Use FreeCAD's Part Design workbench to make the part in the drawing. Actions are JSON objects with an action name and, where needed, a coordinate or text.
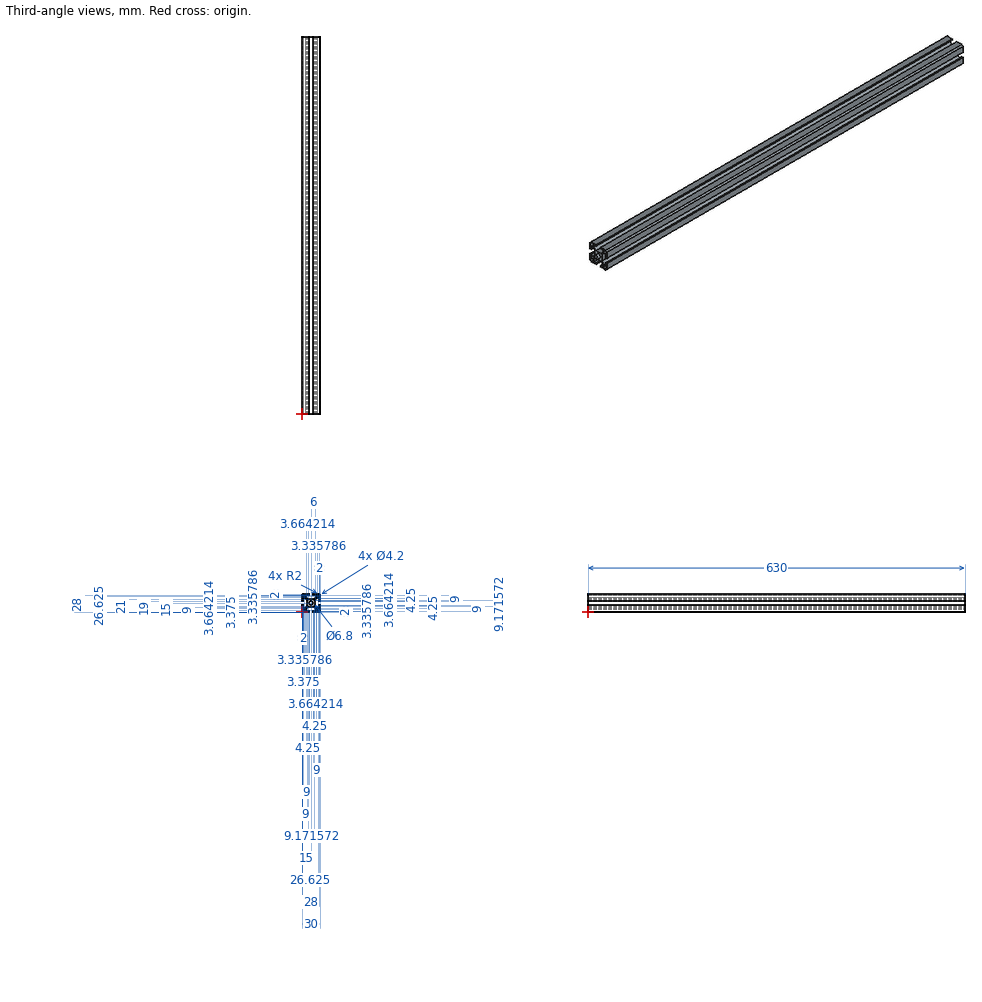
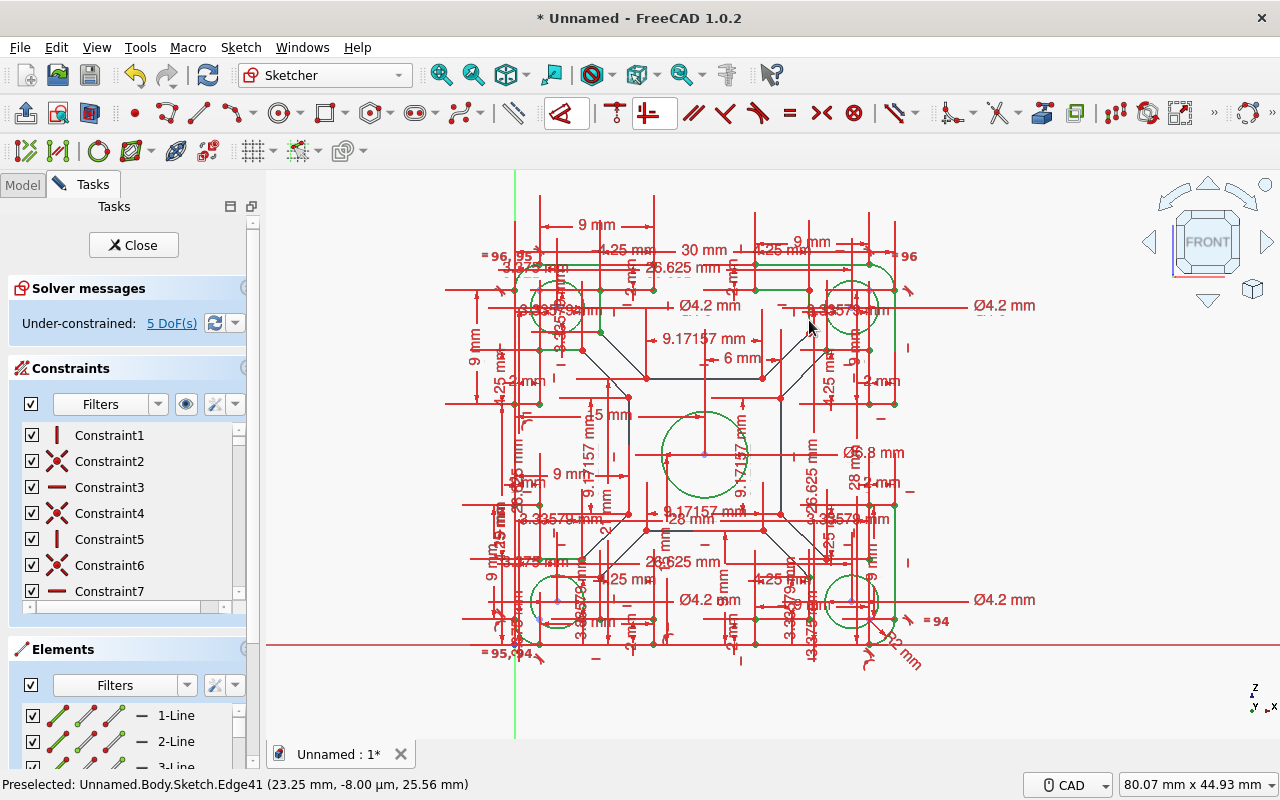
{"action": "left_click", "coordinate": [584, 114]}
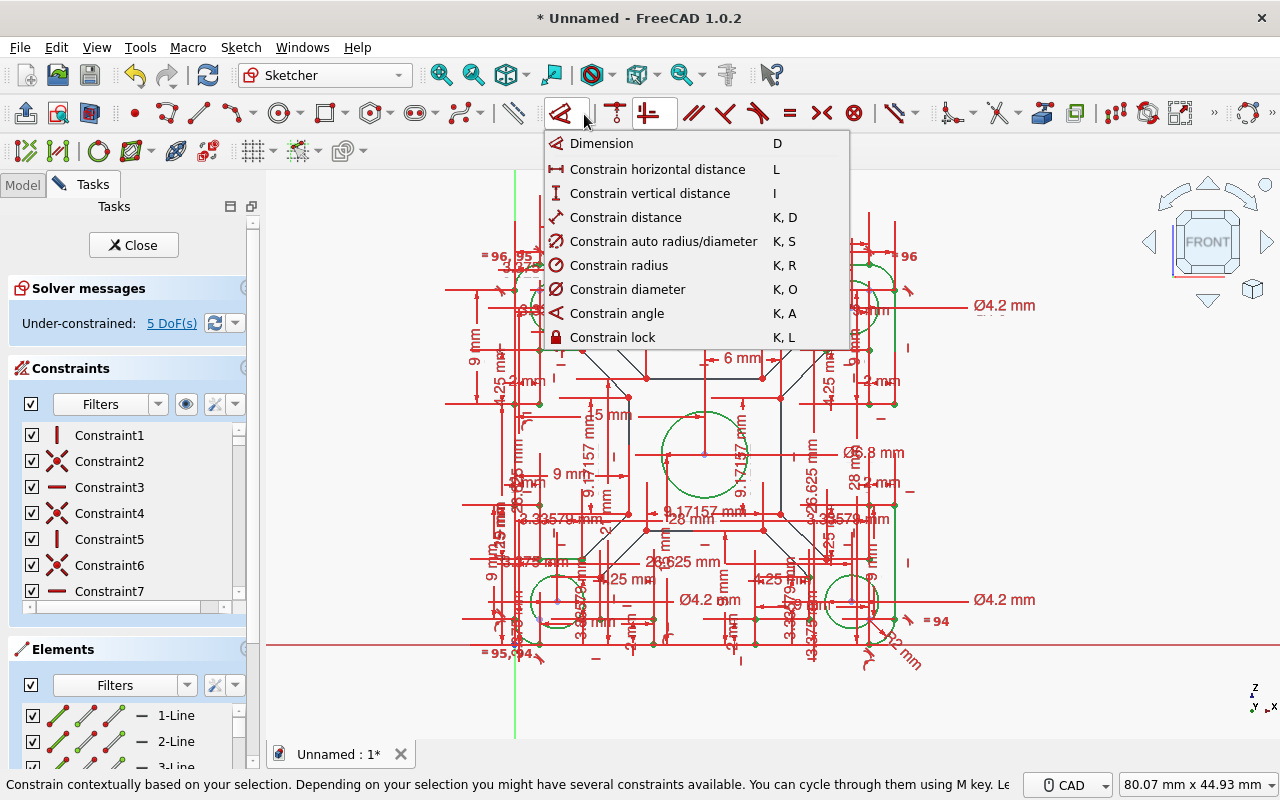
{"action": "left_click", "coordinate": [697, 193]}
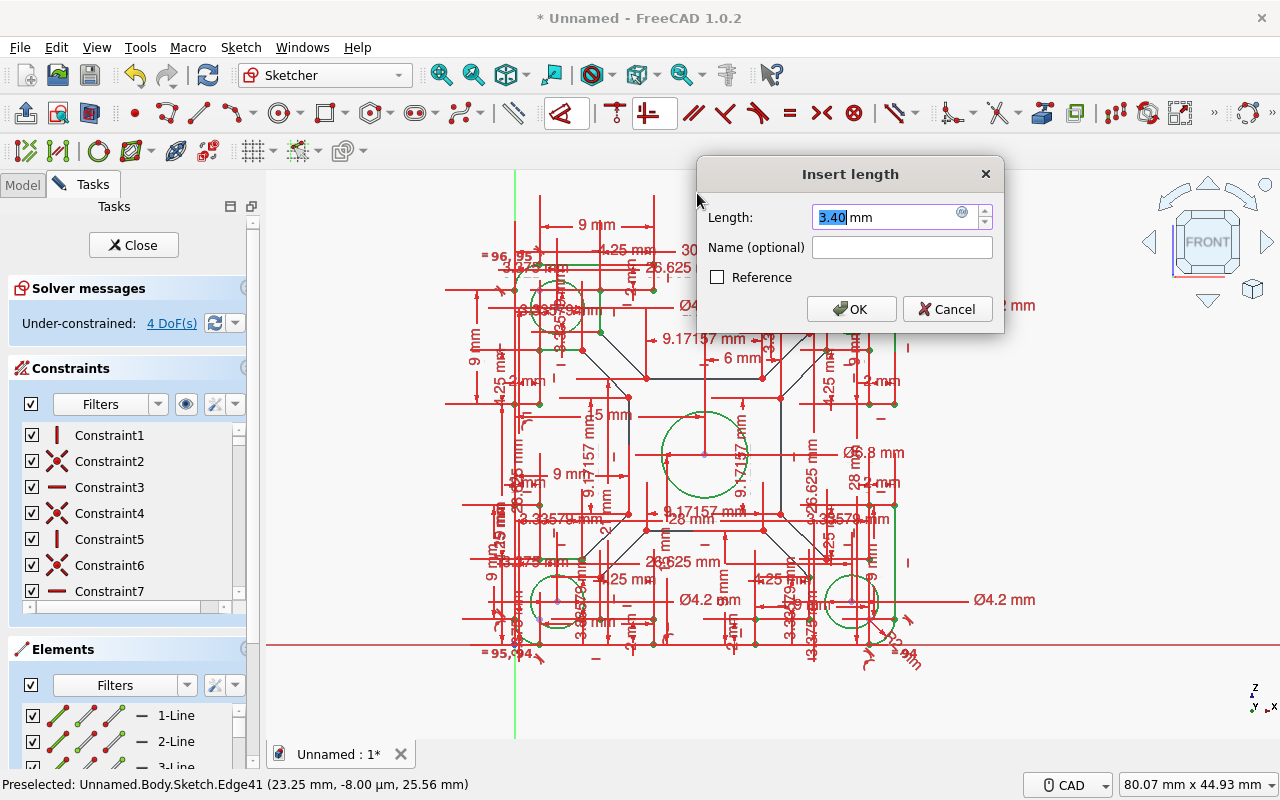
{"action": "type", "text": "3.335786"}
{"action": "key", "text": "Return"}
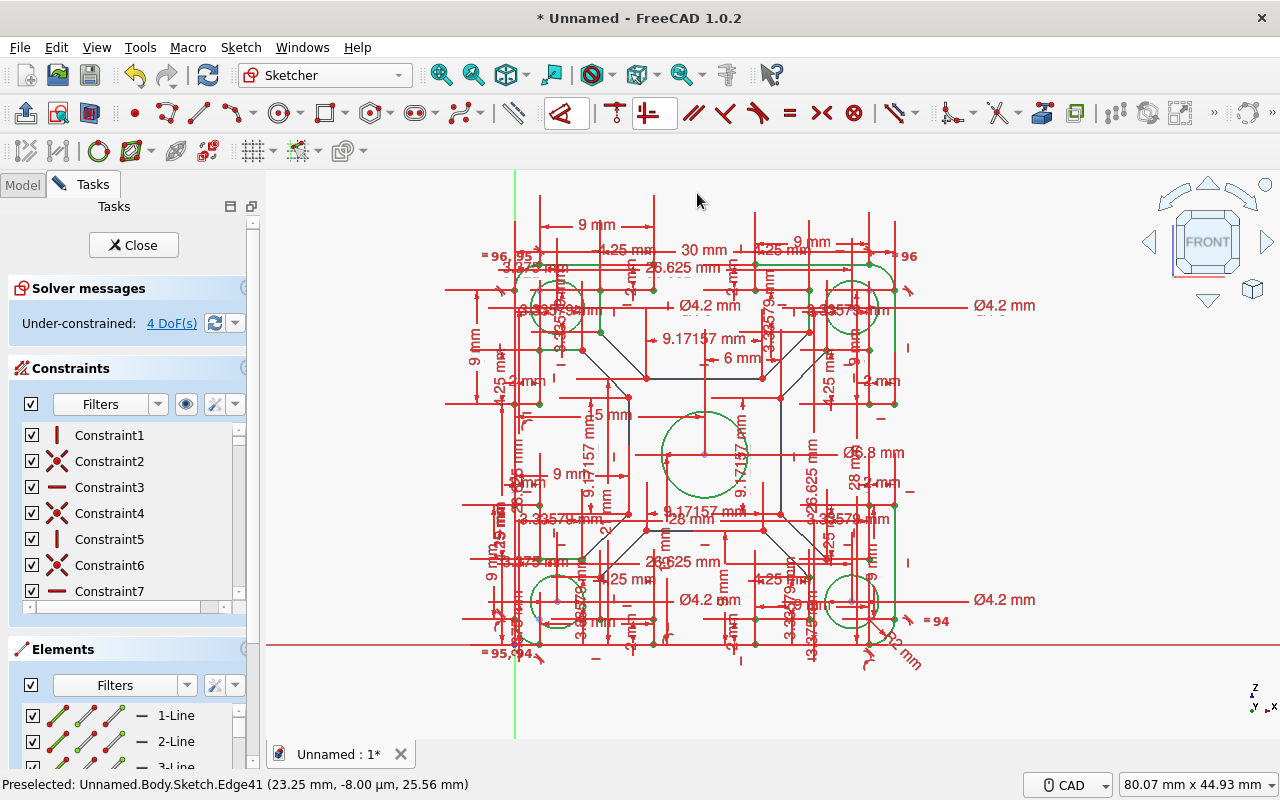
{"action": "left_click", "coordinate": [813, 365]}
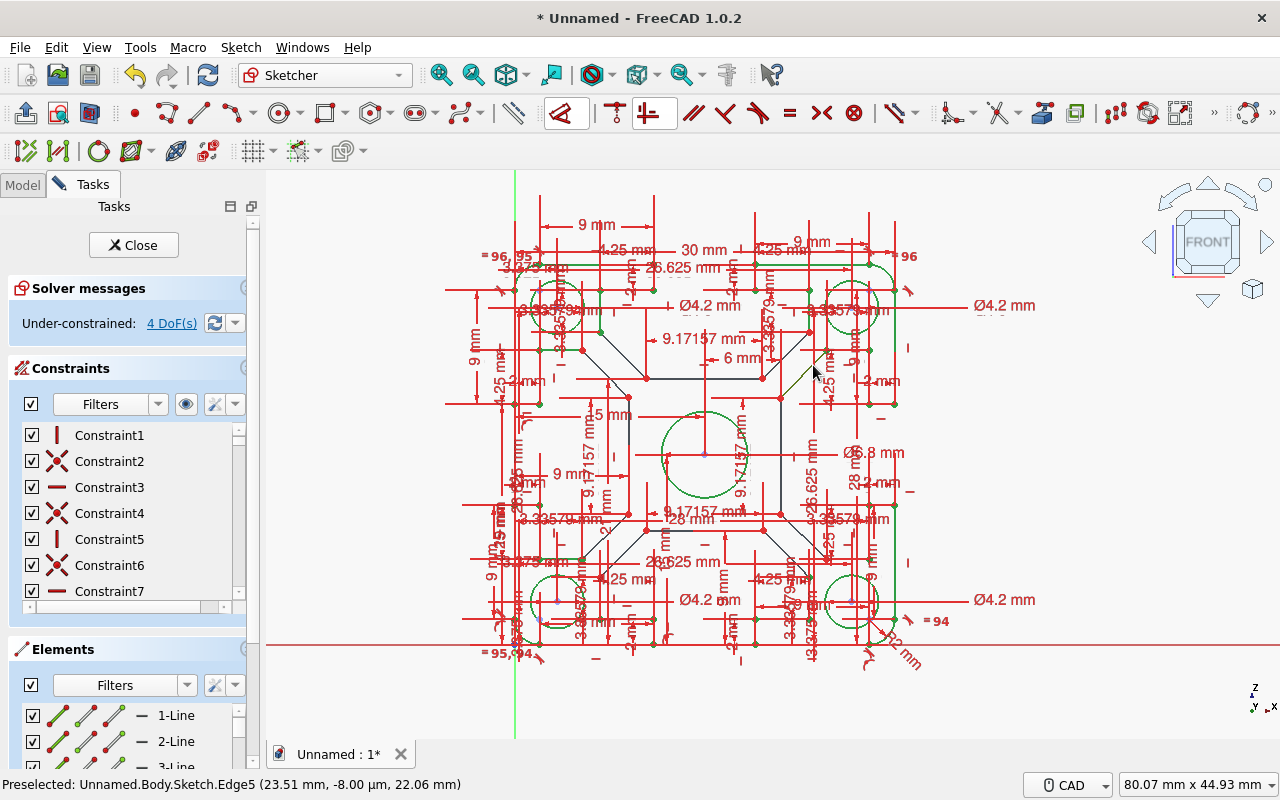
{"action": "left_click", "coordinate": [584, 114]}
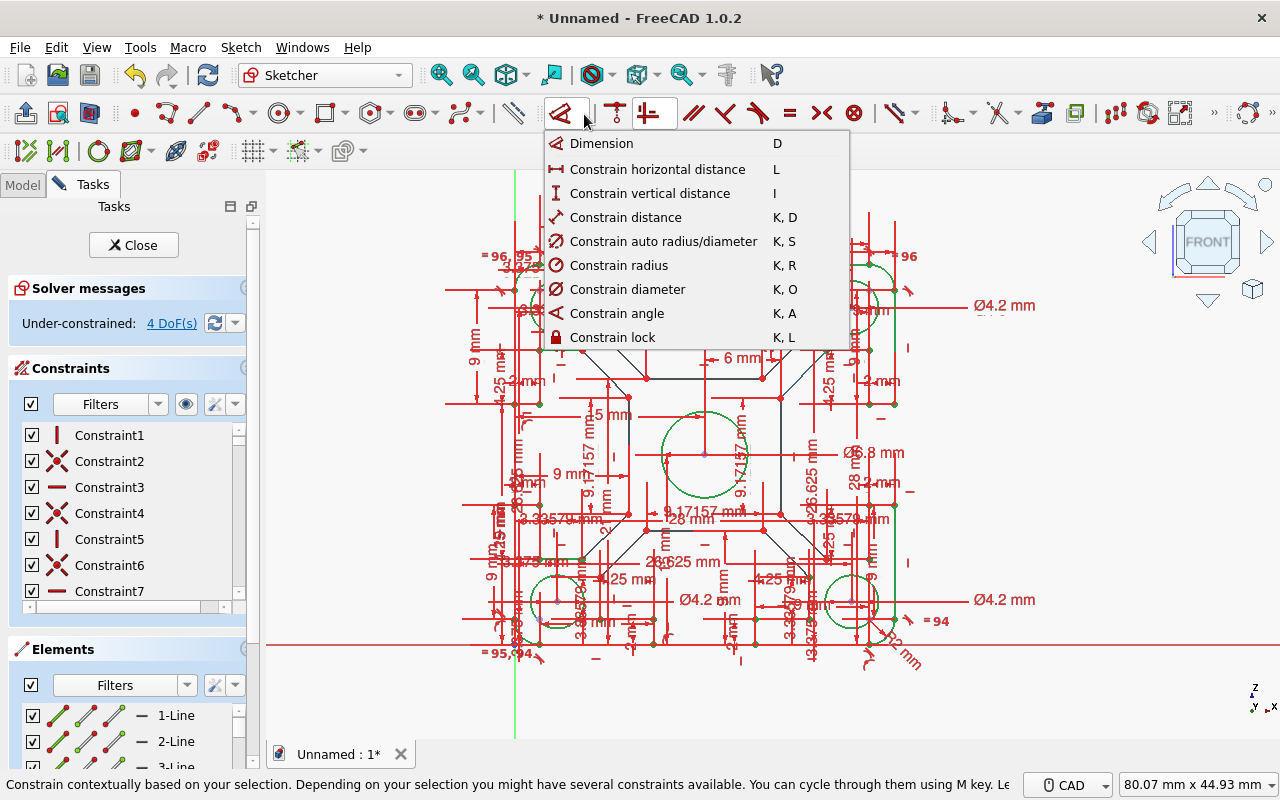
{"action": "left_click", "coordinate": [697, 193]}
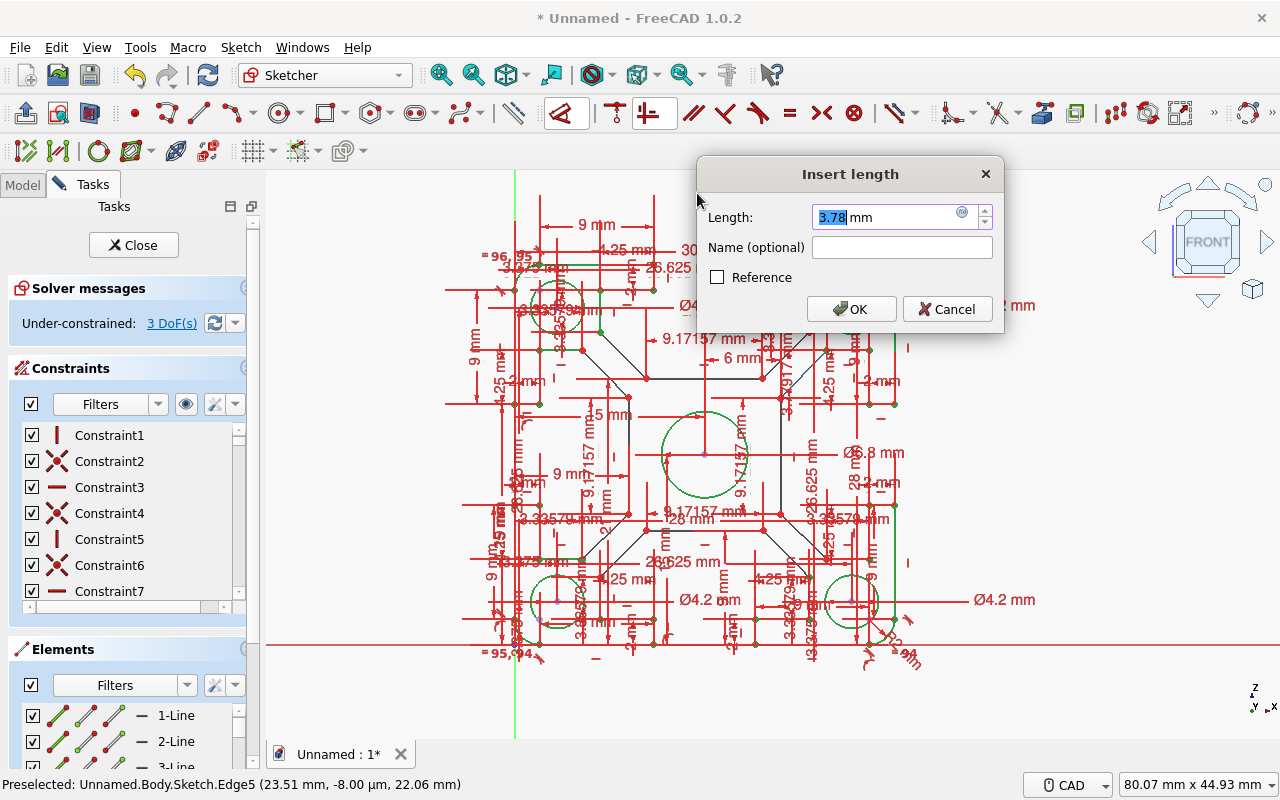
{"action": "type", "text": "3.664214"}
{"action": "key", "text": "Return"}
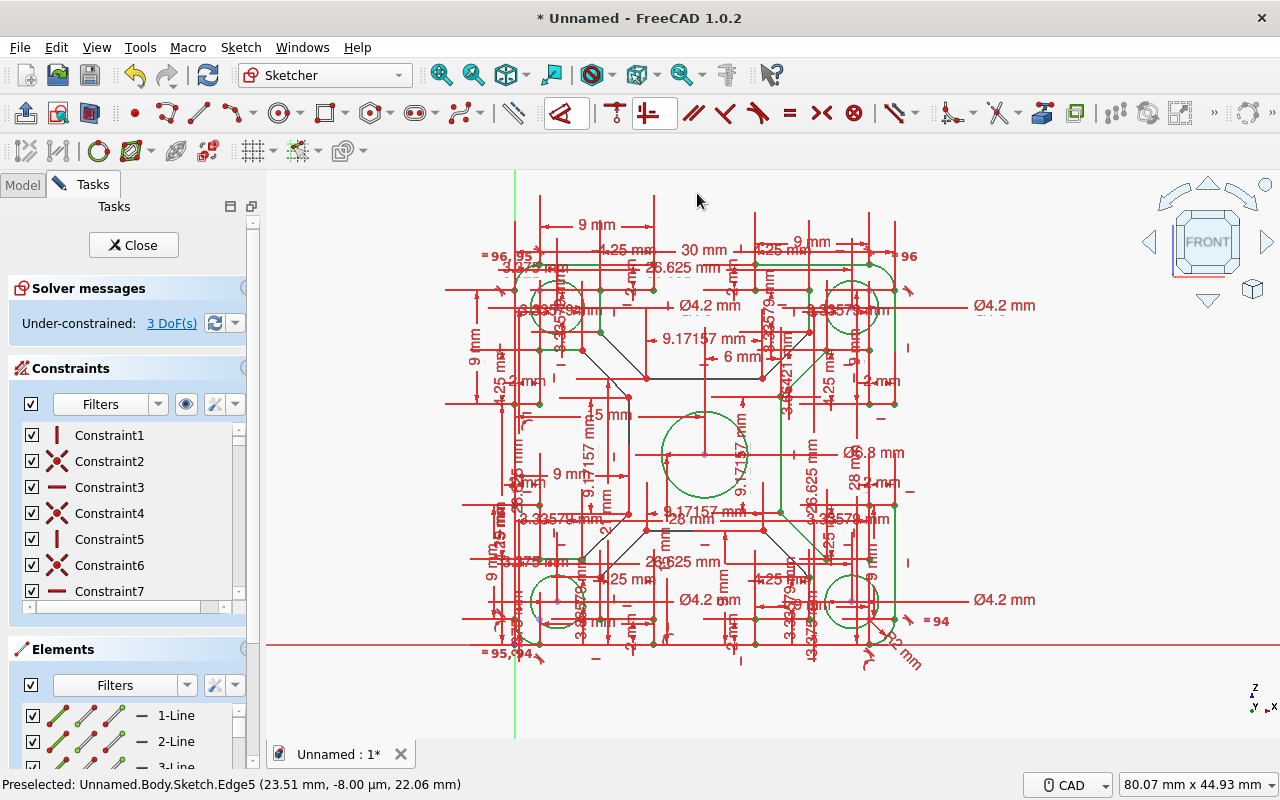
{"action": "left_click", "coordinate": [777, 545]}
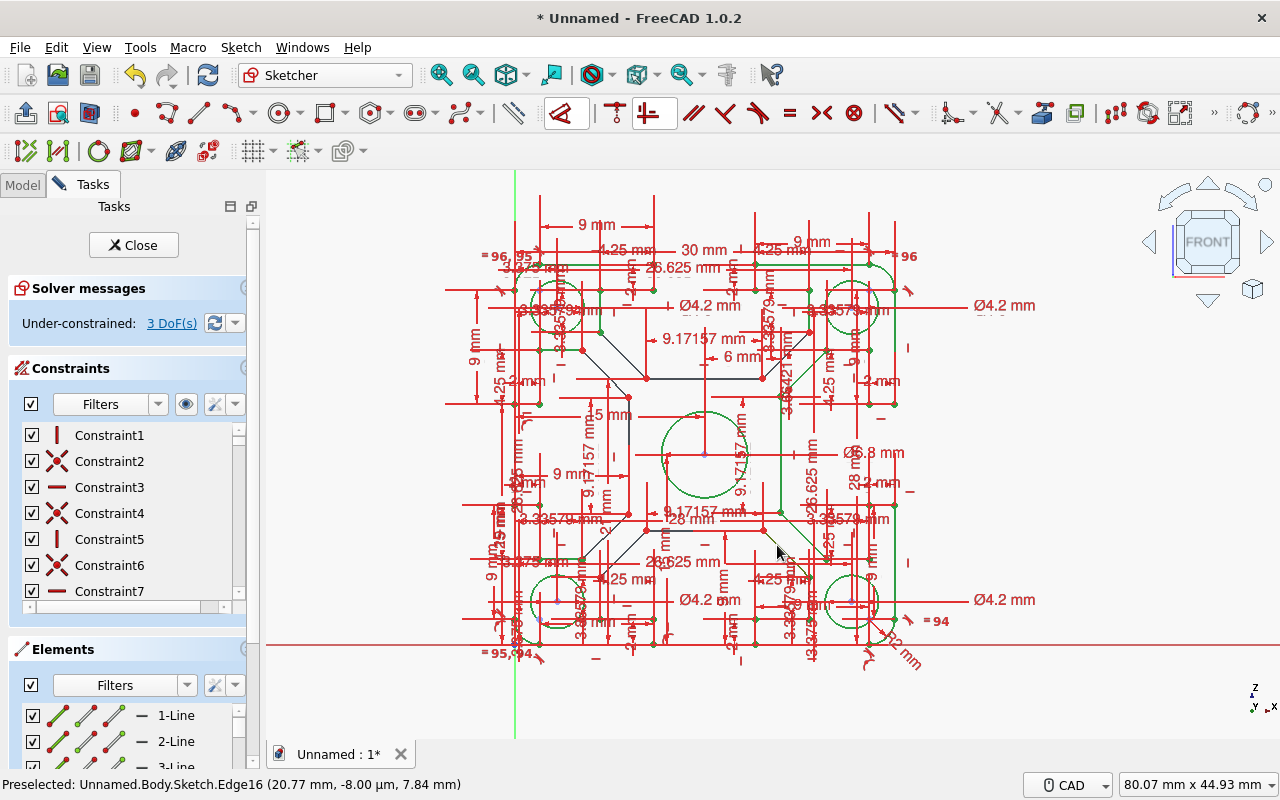
{"action": "key", "text": "l"}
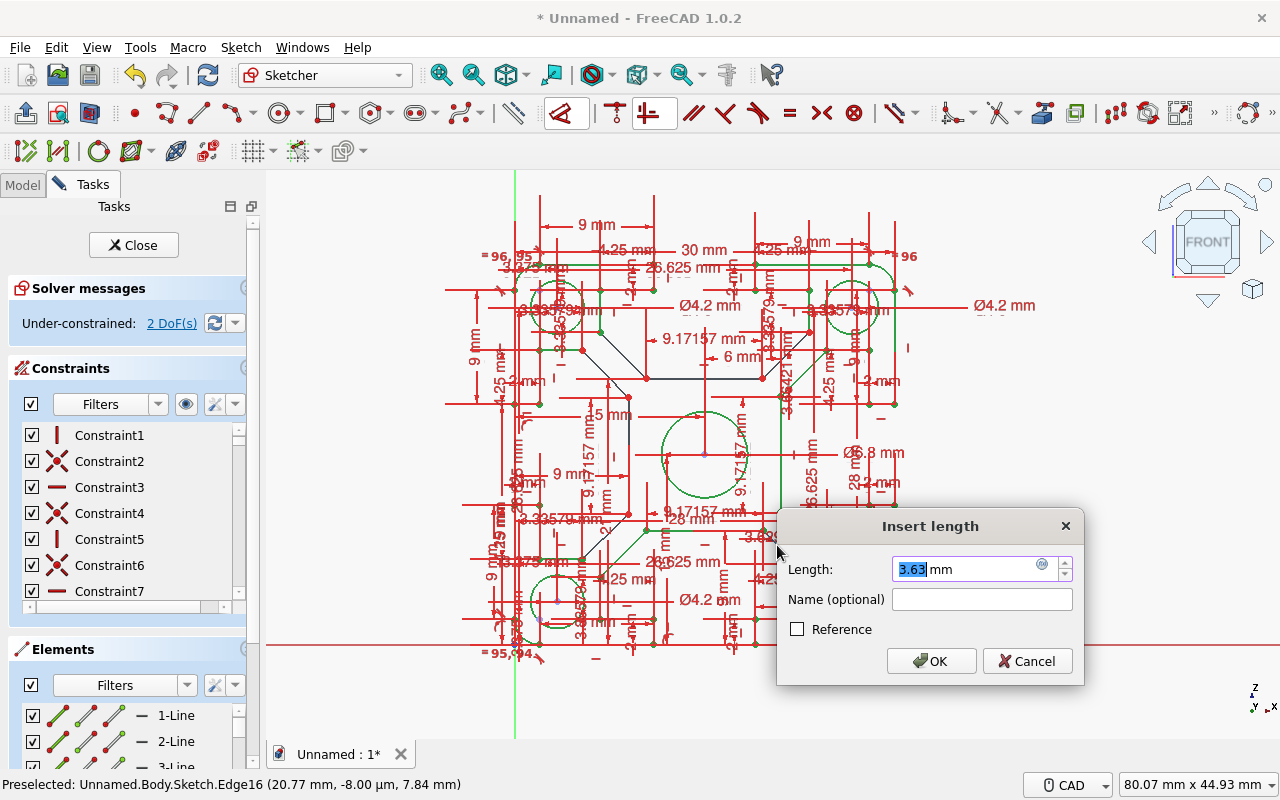
{"action": "type", "text": "3.664214"}
{"action": "key", "text": "Return"}